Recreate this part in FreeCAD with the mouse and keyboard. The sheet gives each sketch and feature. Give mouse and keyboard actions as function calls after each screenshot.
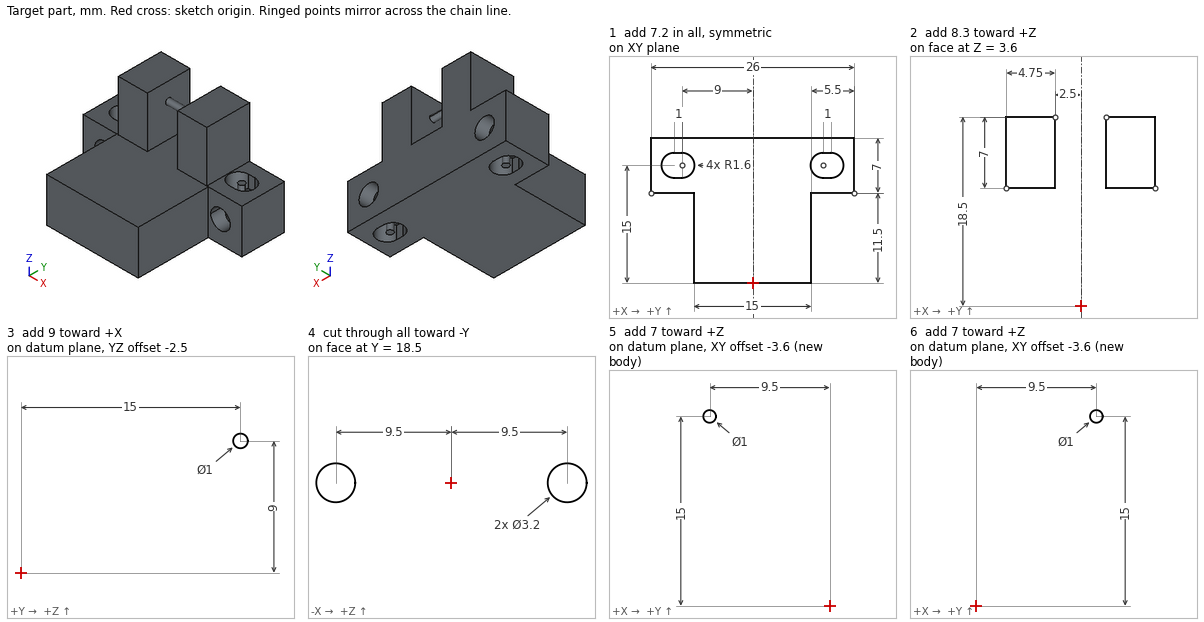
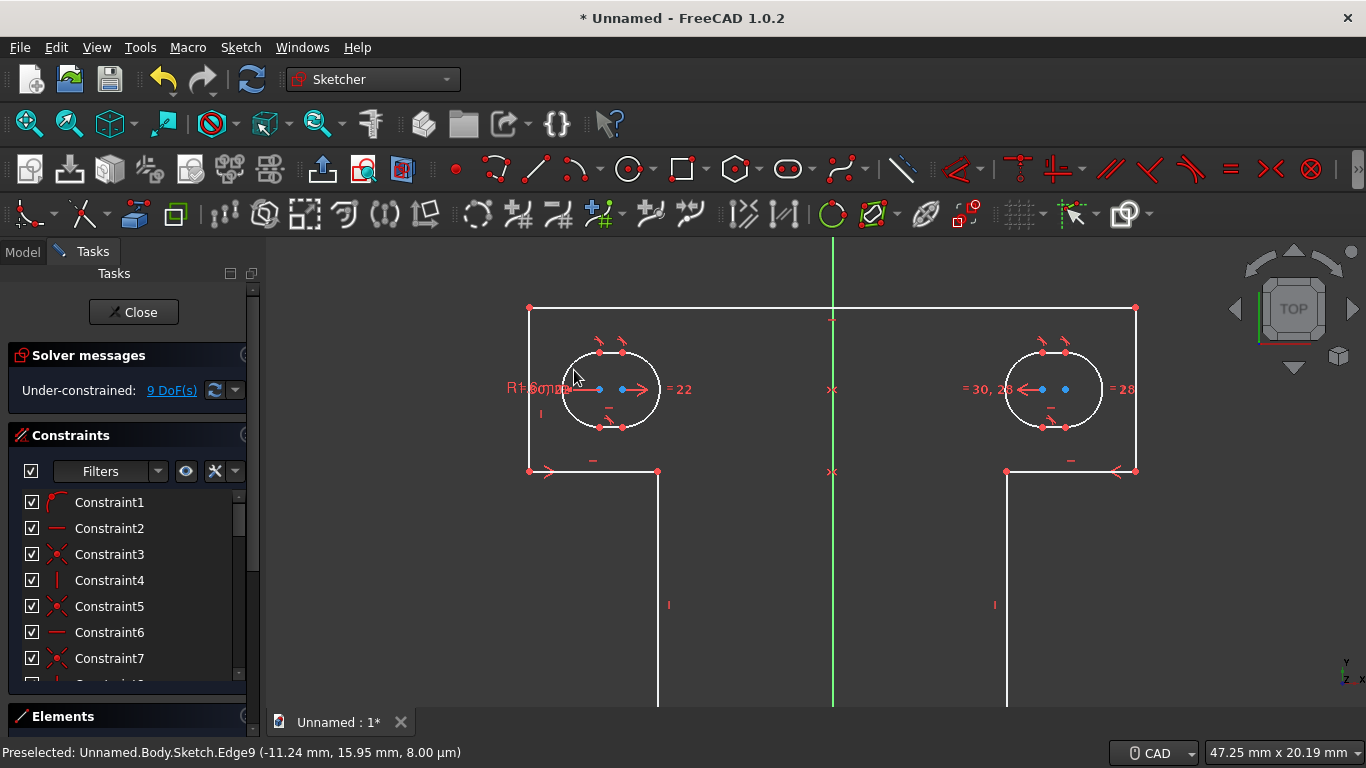
click(951, 405)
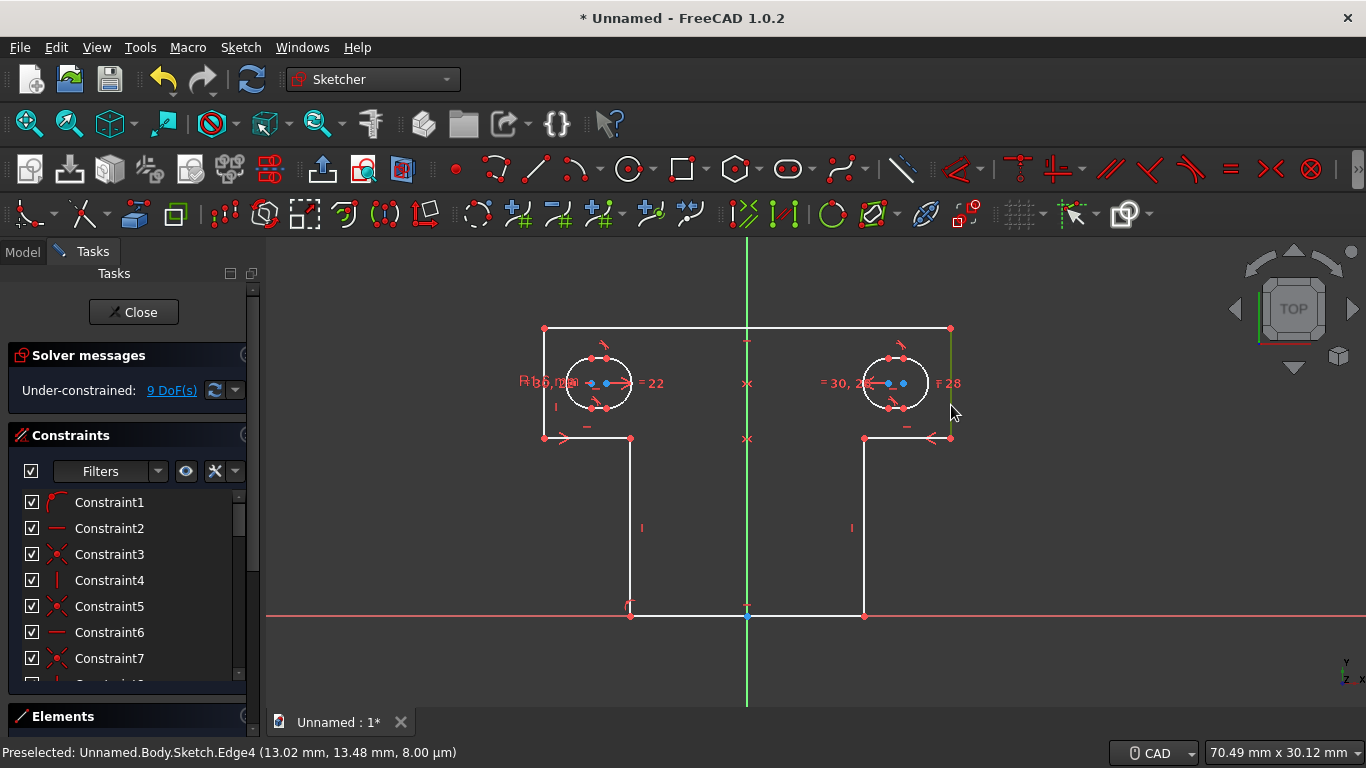
key(i)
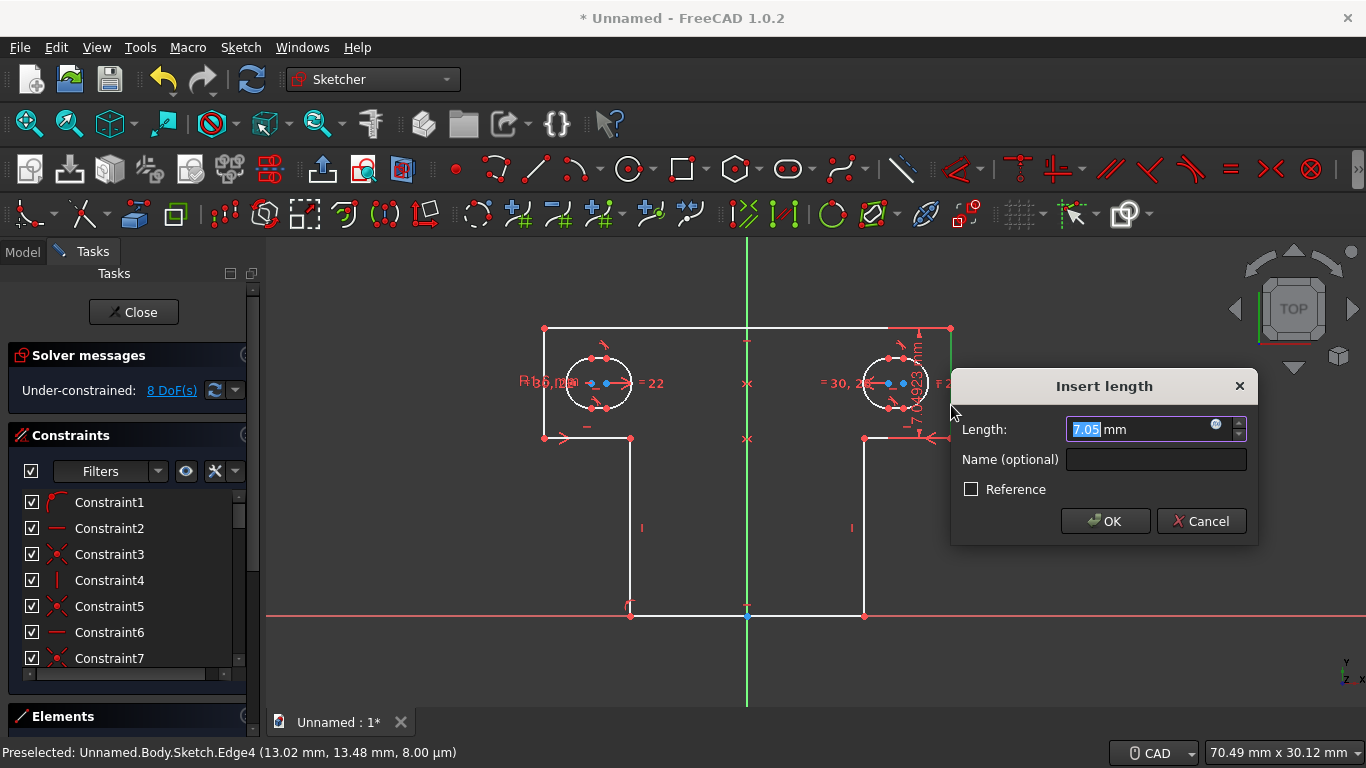
text(7)
key(Return)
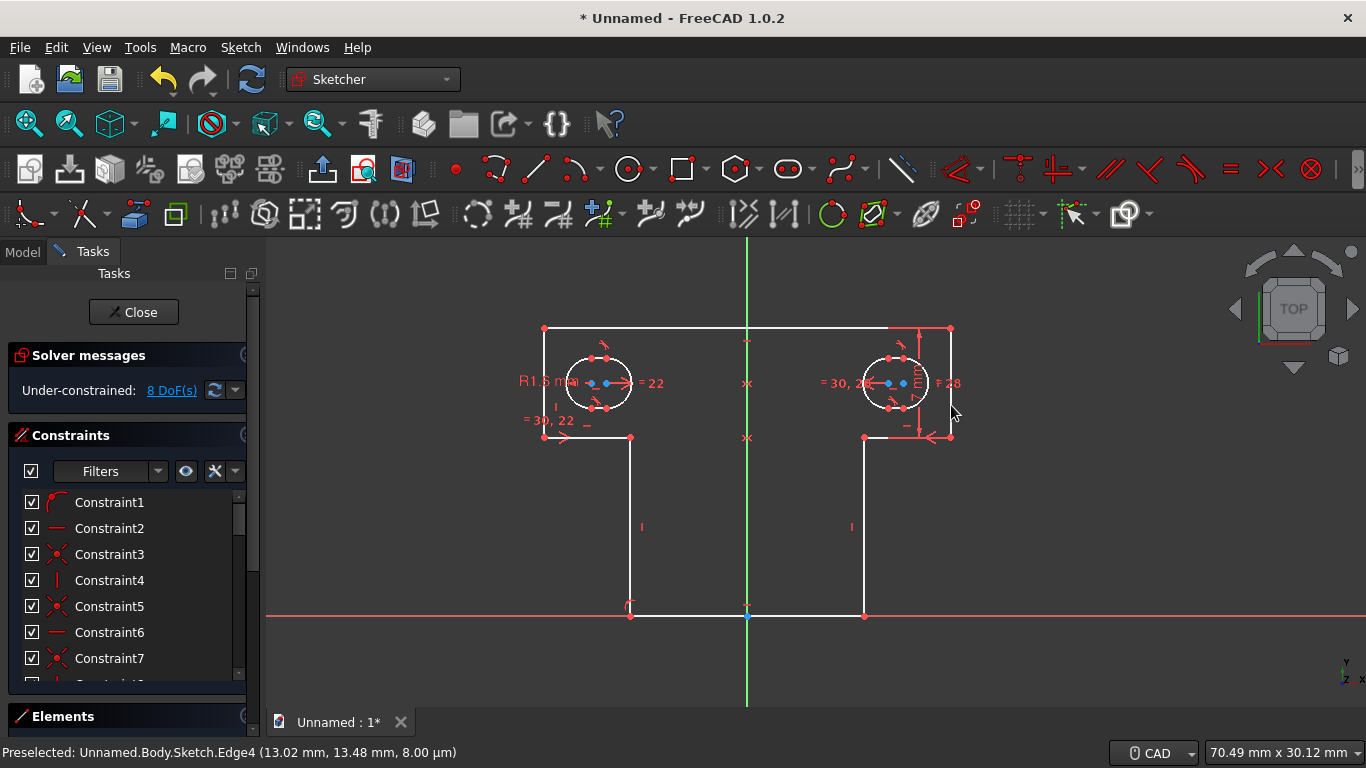
scroll(599, 358, up, 5)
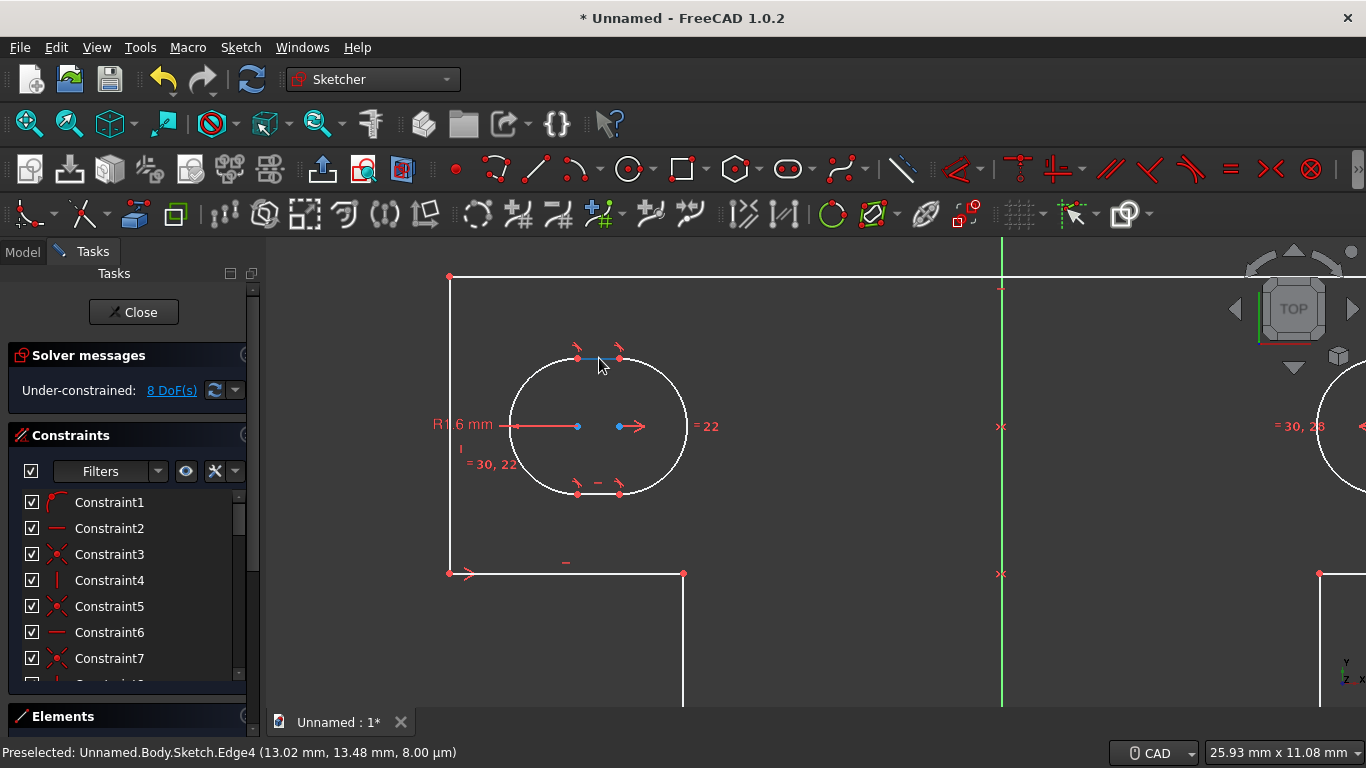
click(598, 359)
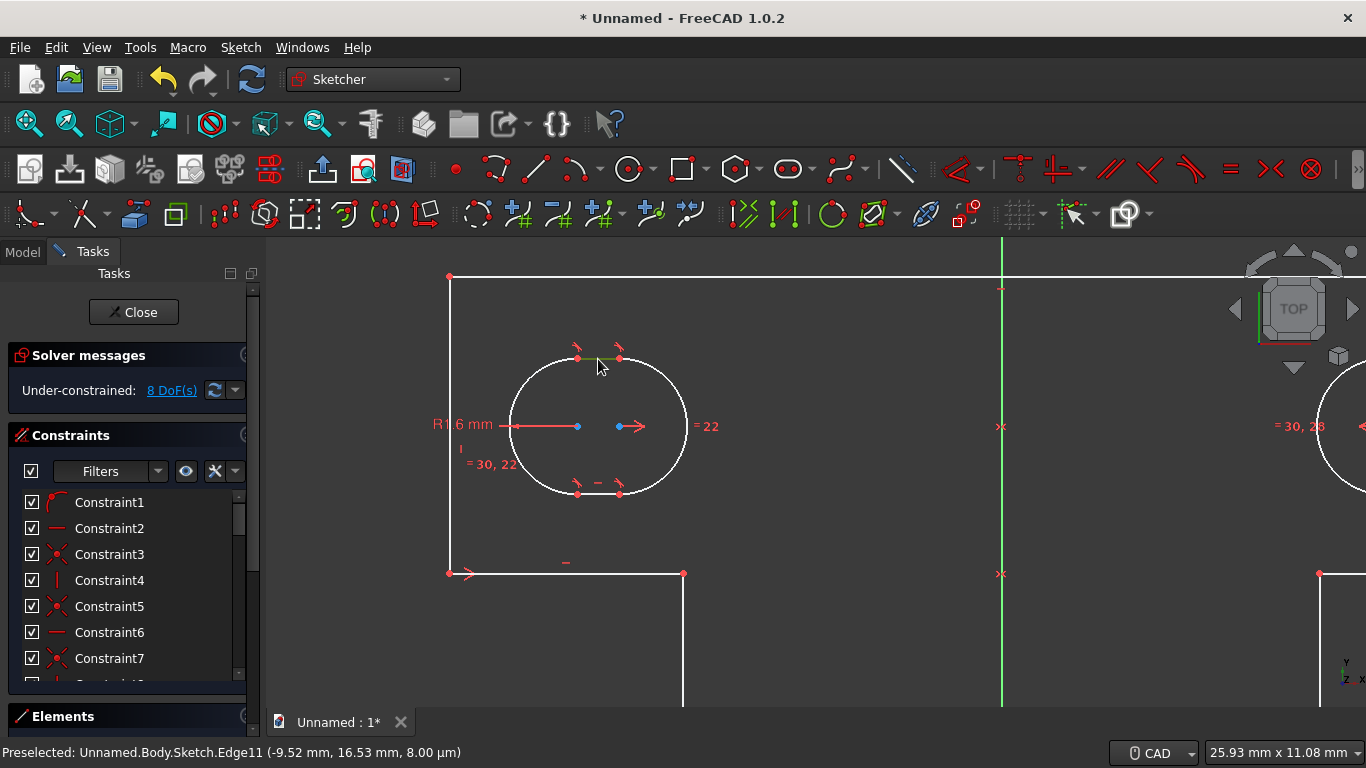
key(l)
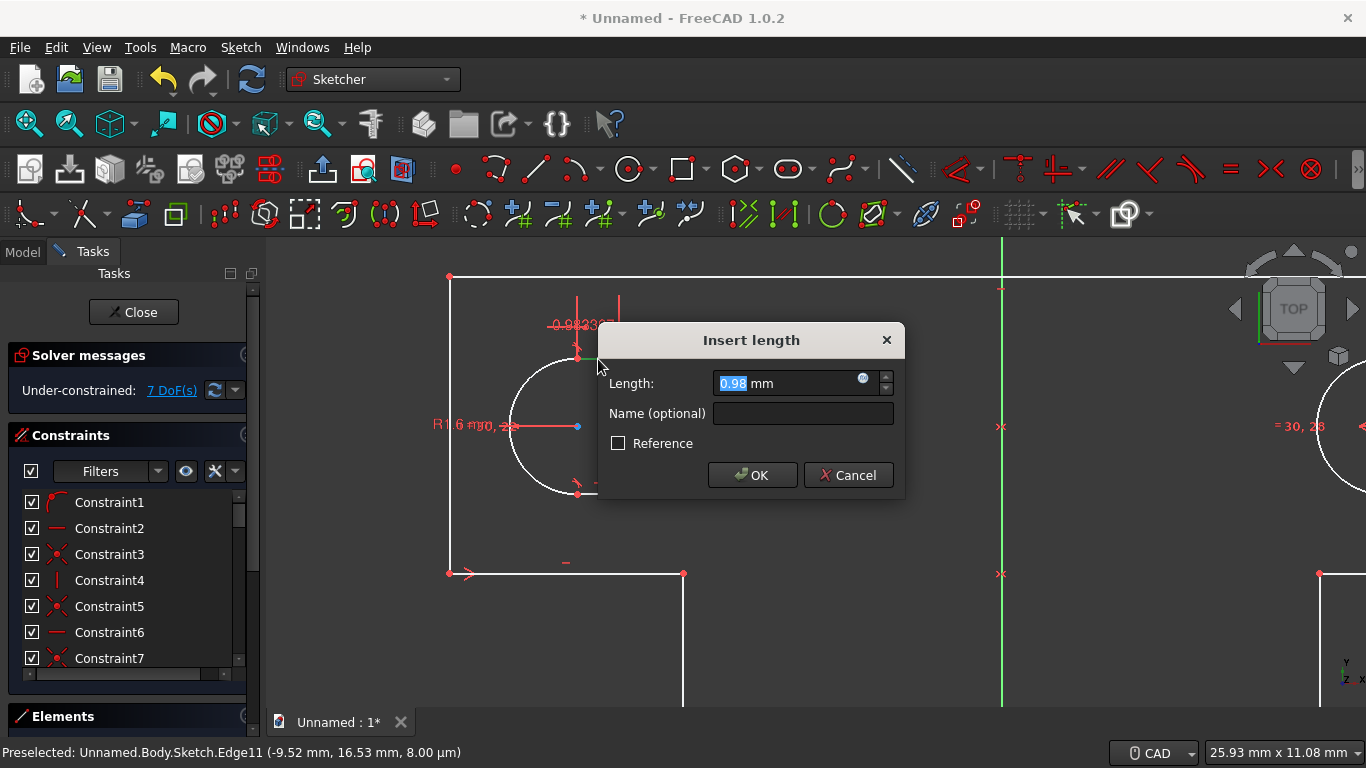
text(1)
key(Return)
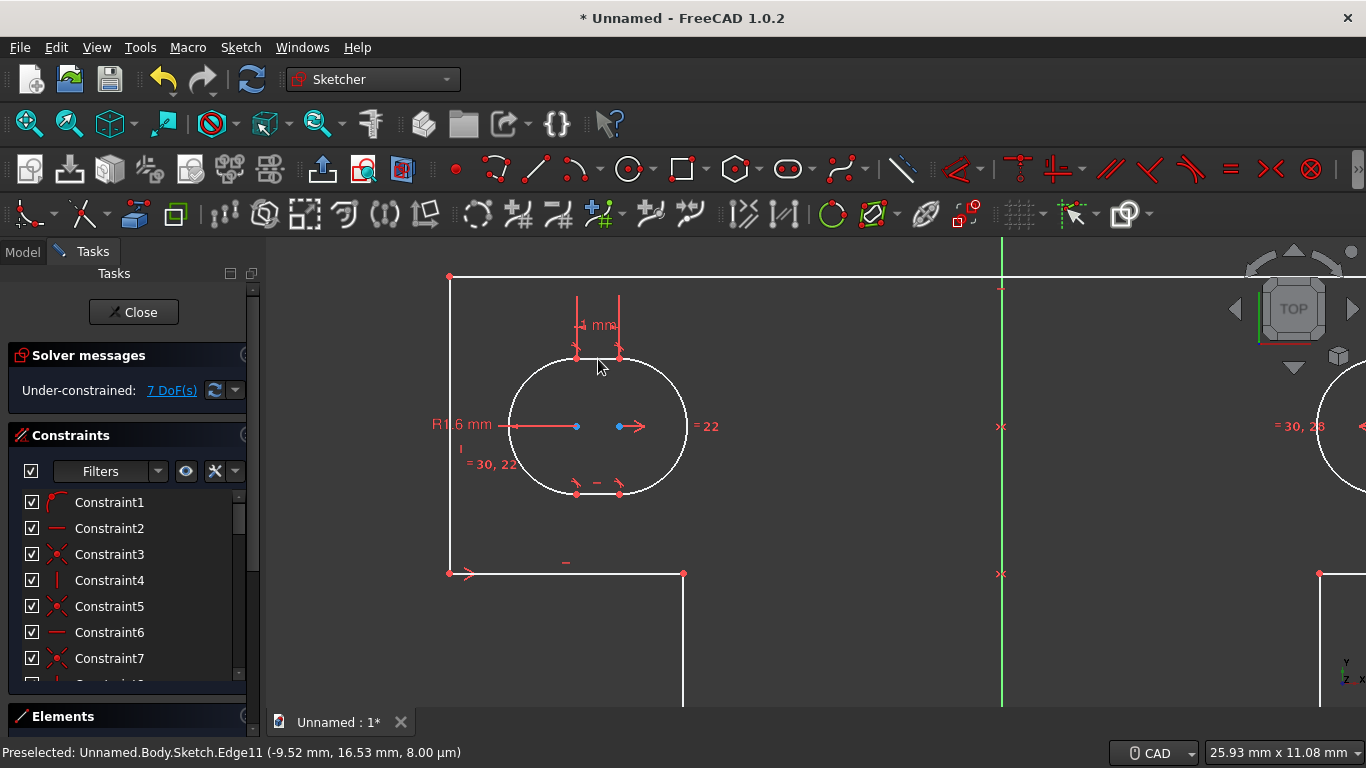
scroll(599, 358, down, 5)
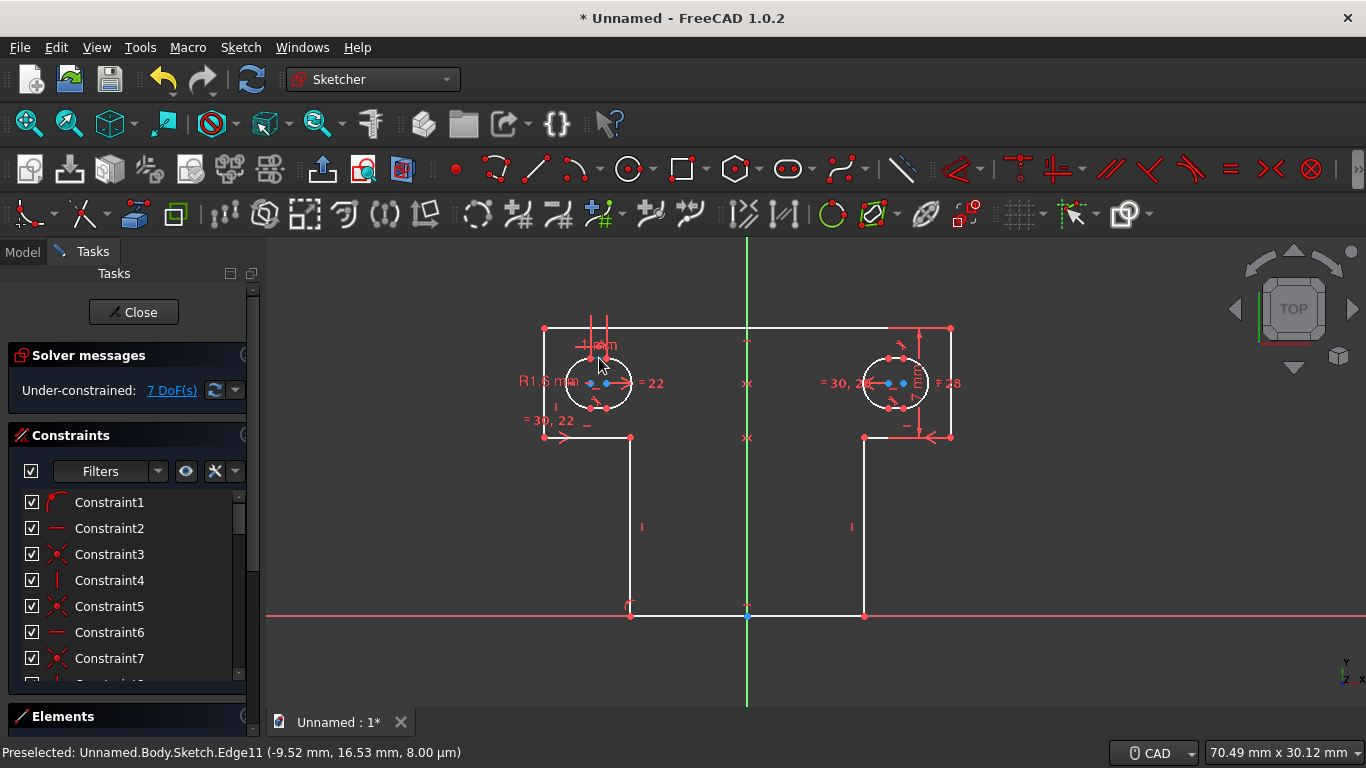
scroll(893, 358, up, 6)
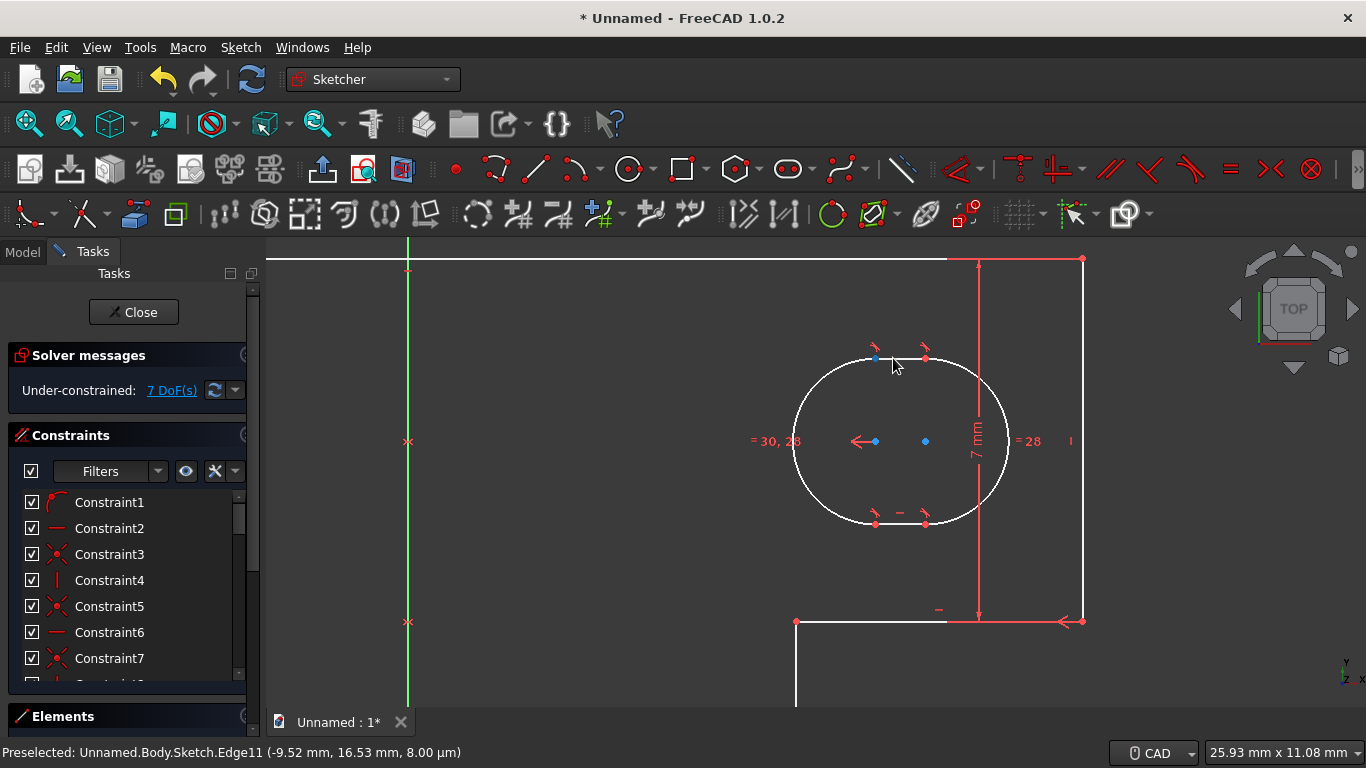
click(891, 359)